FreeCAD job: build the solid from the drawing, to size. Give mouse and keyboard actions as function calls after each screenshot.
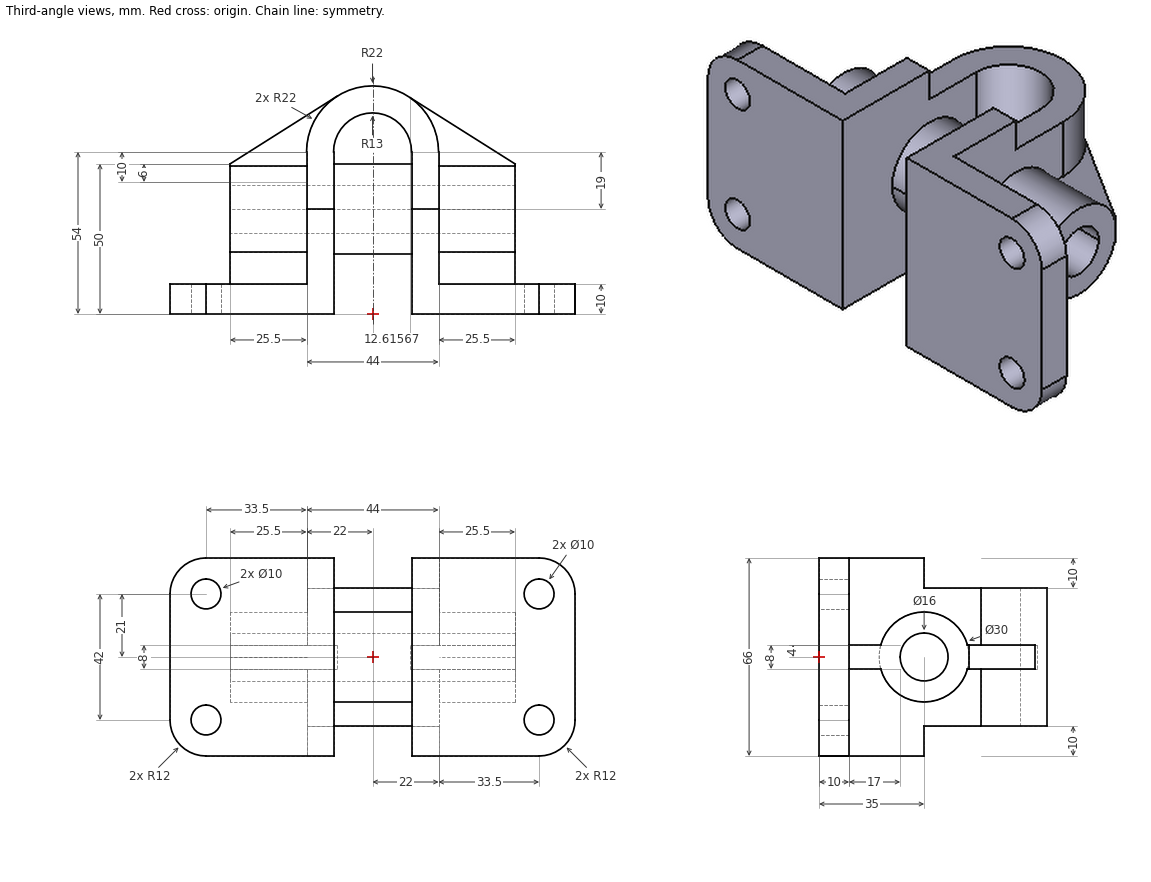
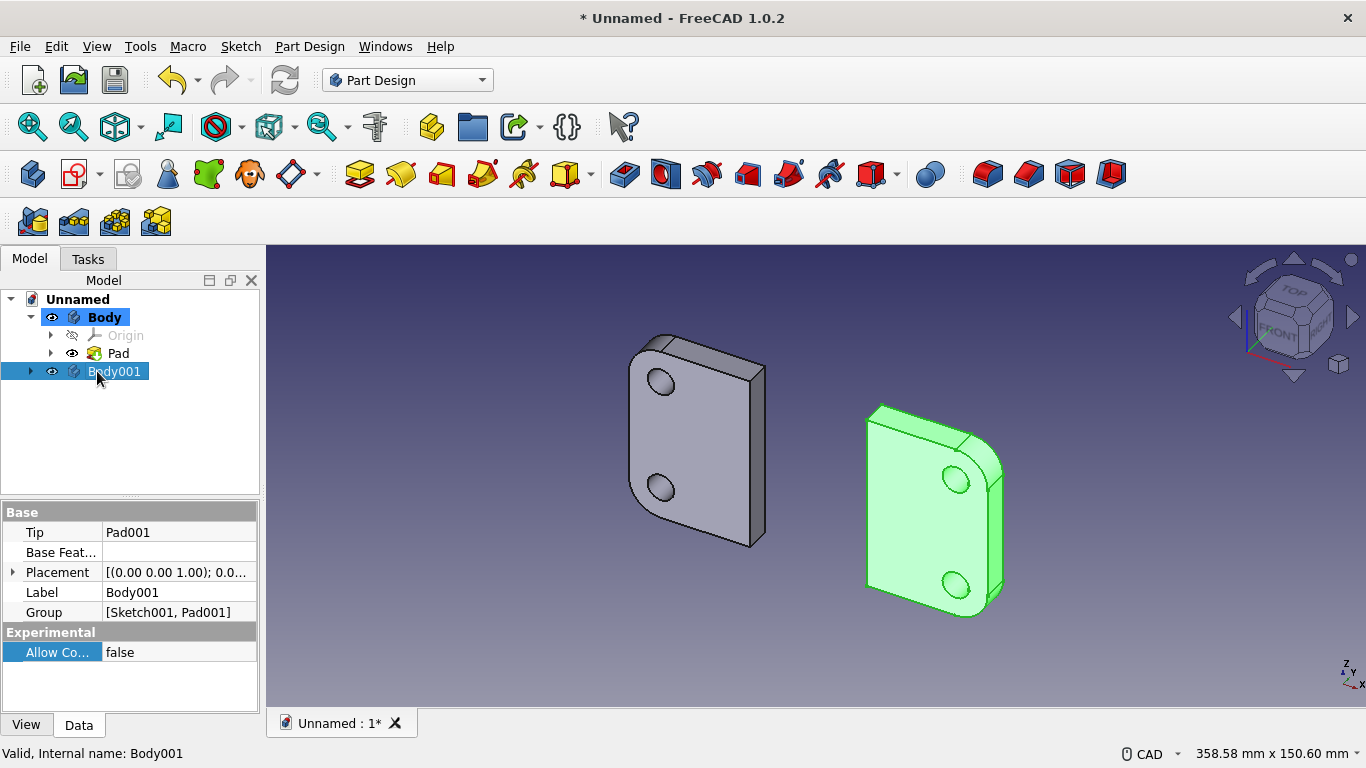
click(931, 174)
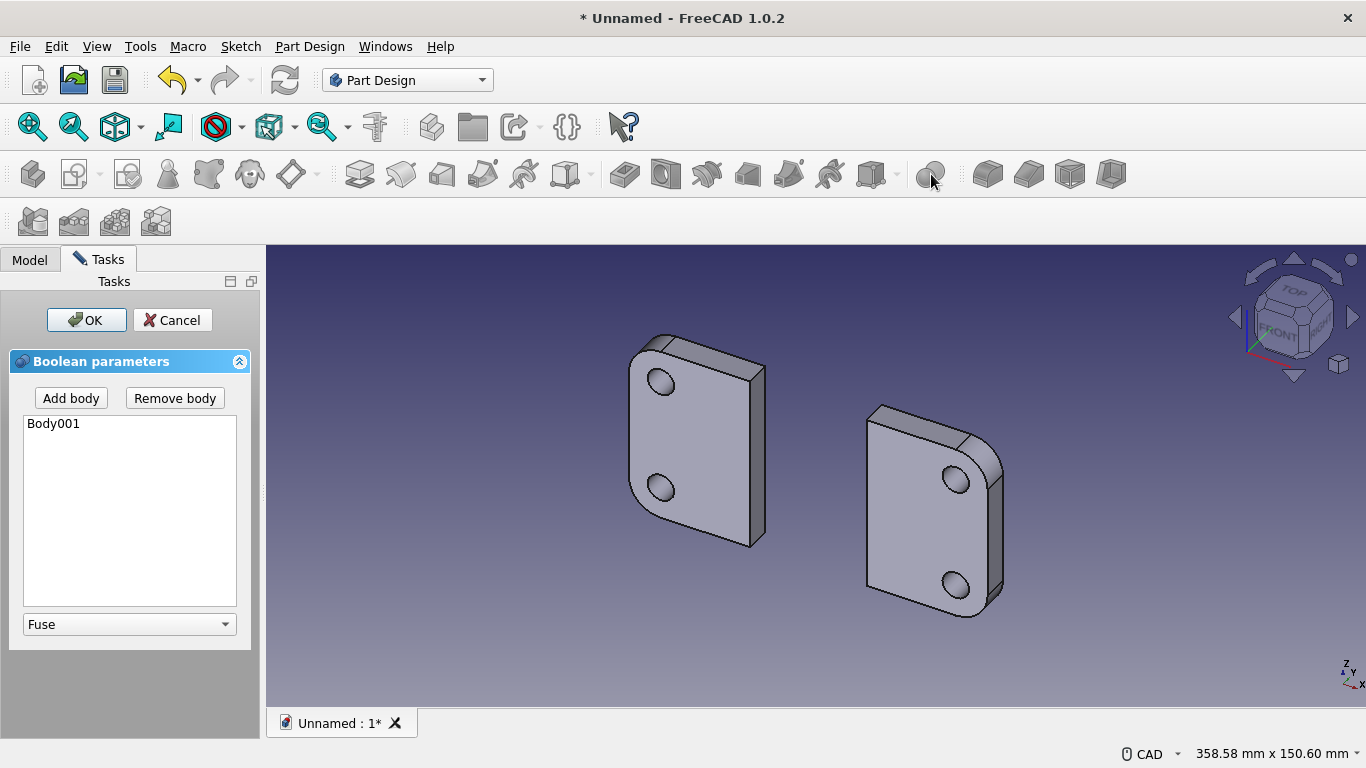
click(87, 320)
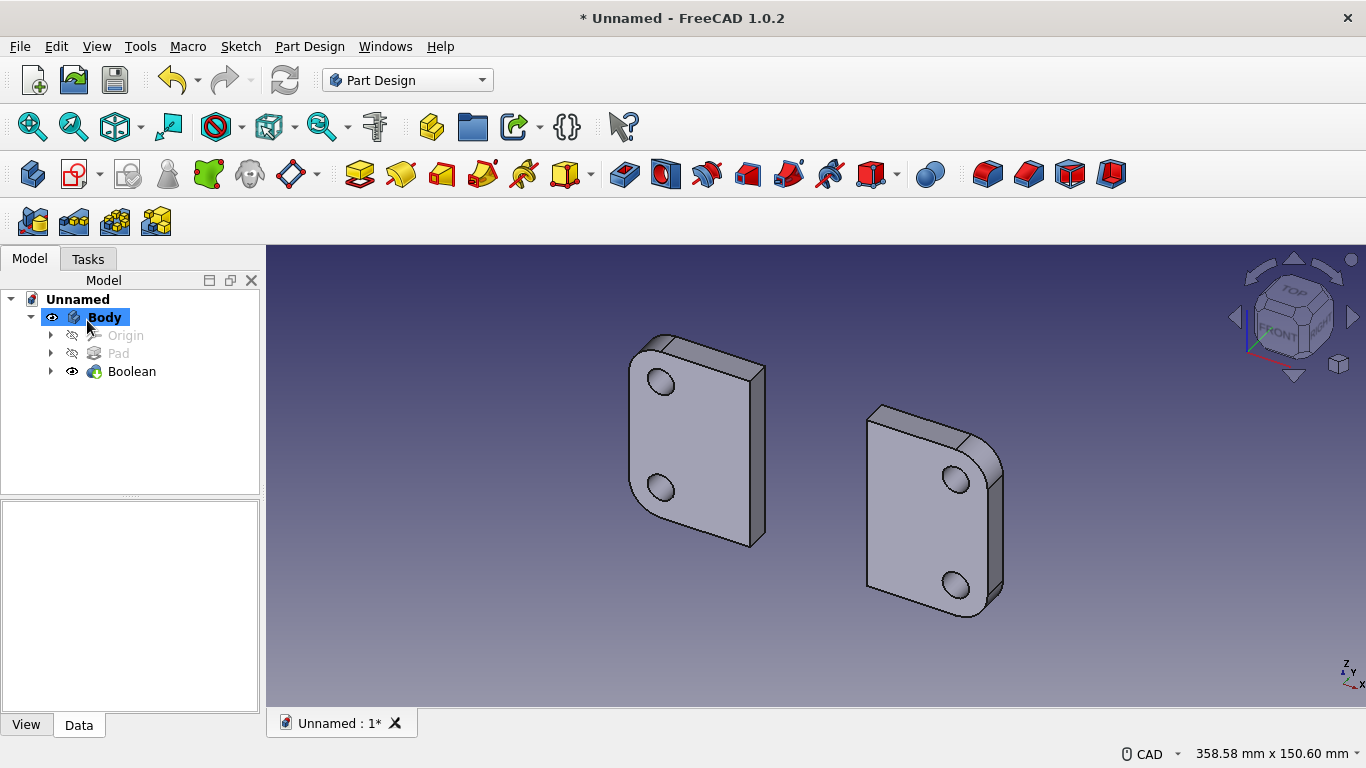
click(738, 366)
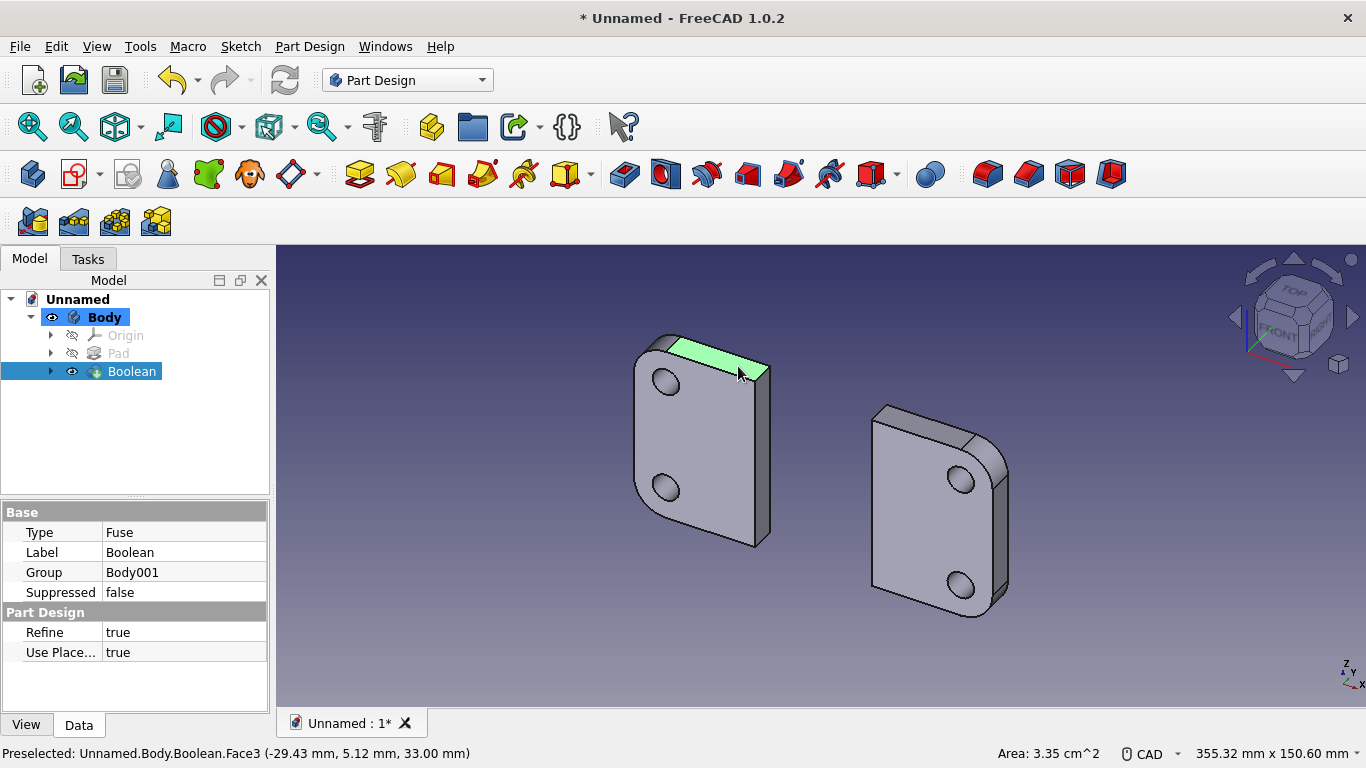
click(74, 174)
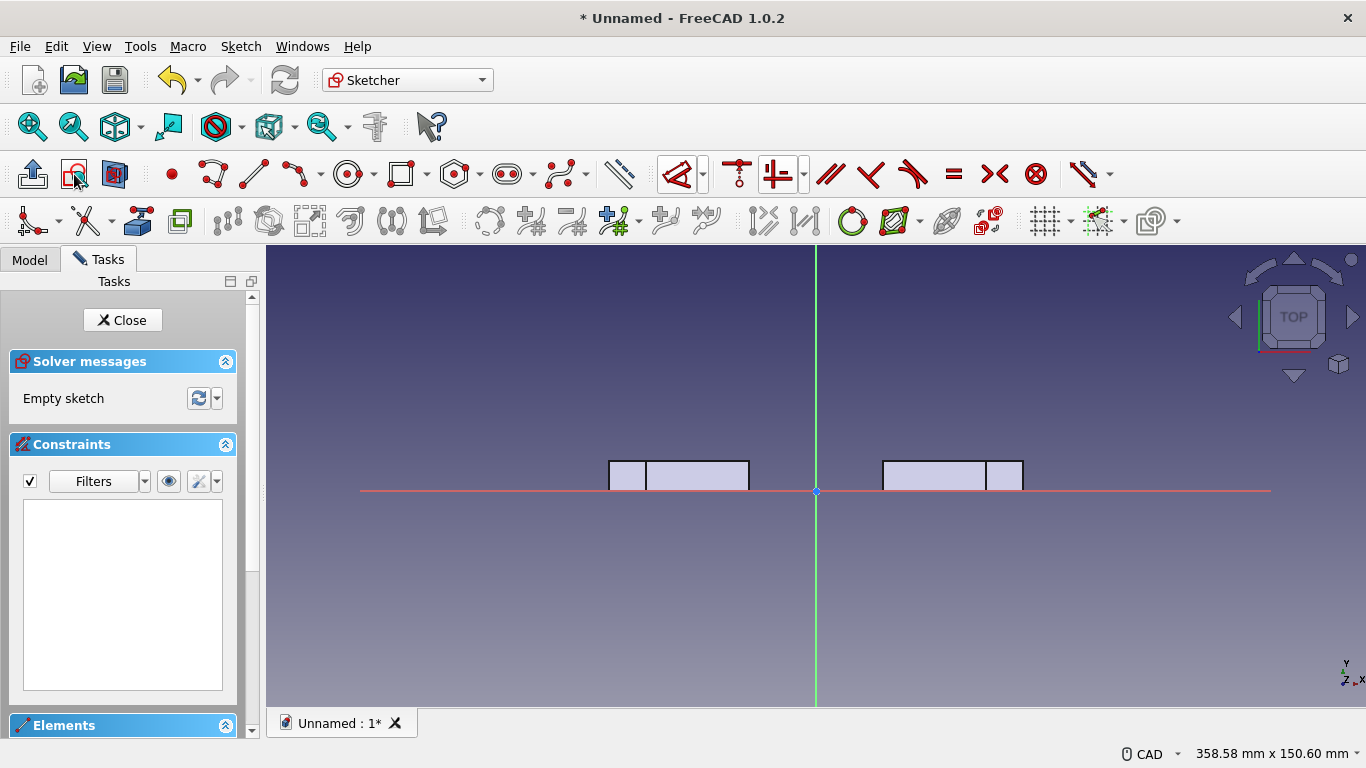
scroll(438, 679, down, 1)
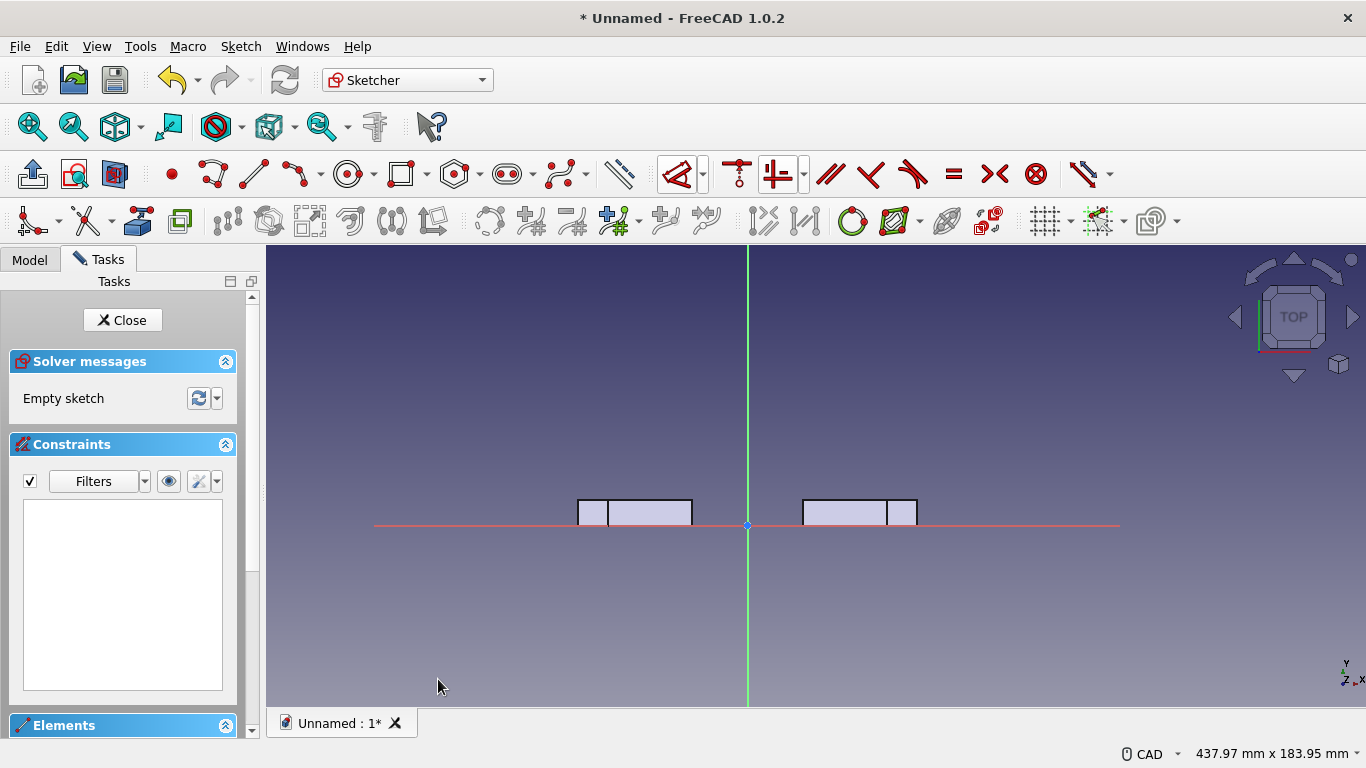
scroll(748, 337, up, 2)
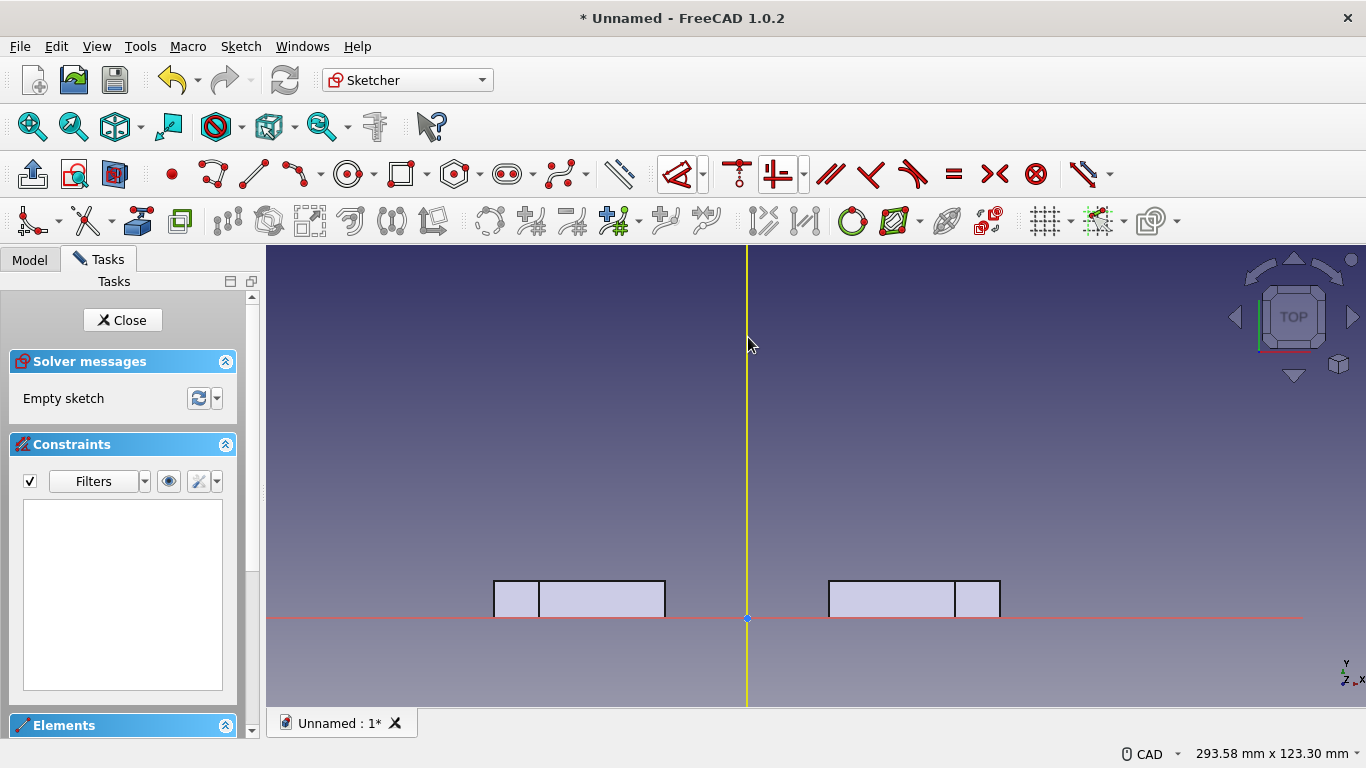
click(213, 174)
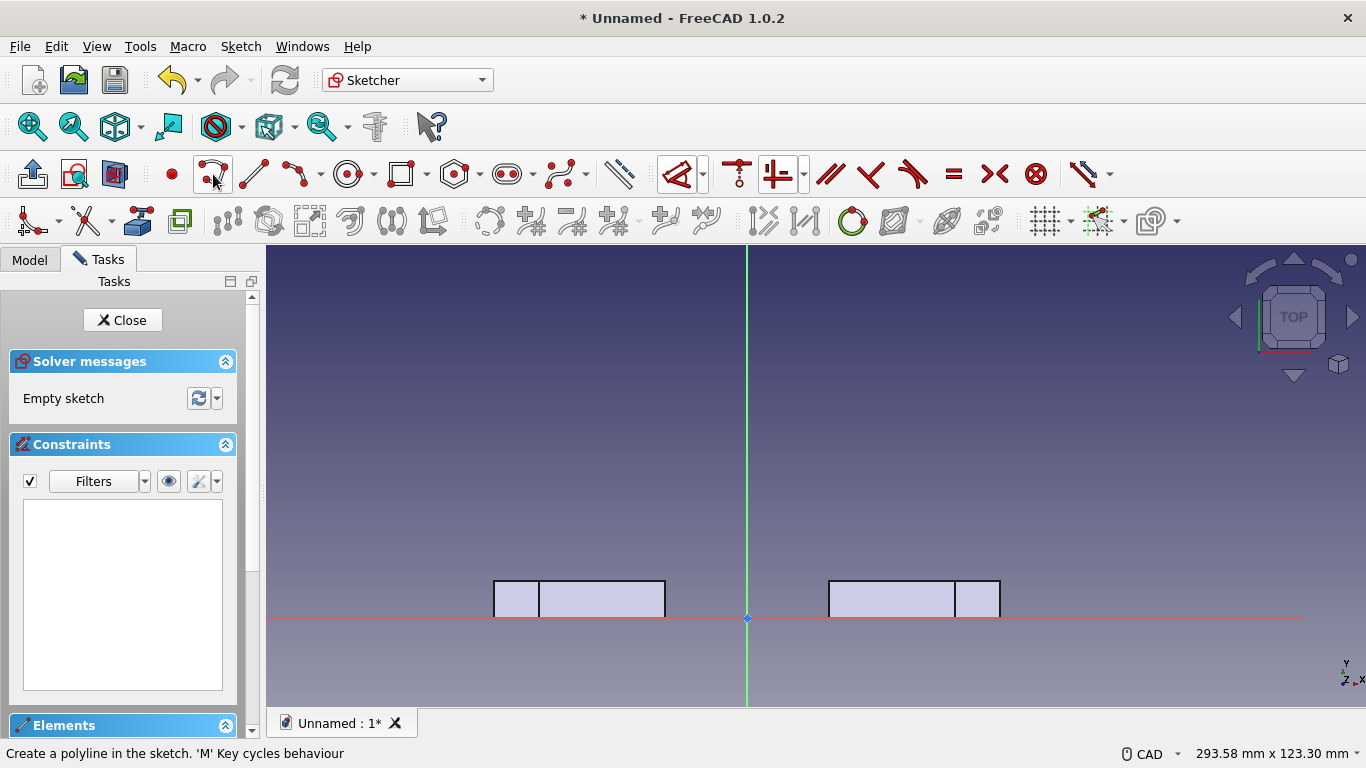
click(665, 416)
click(665, 618)
click(698, 609)
click(698, 416)
right_click(698, 416)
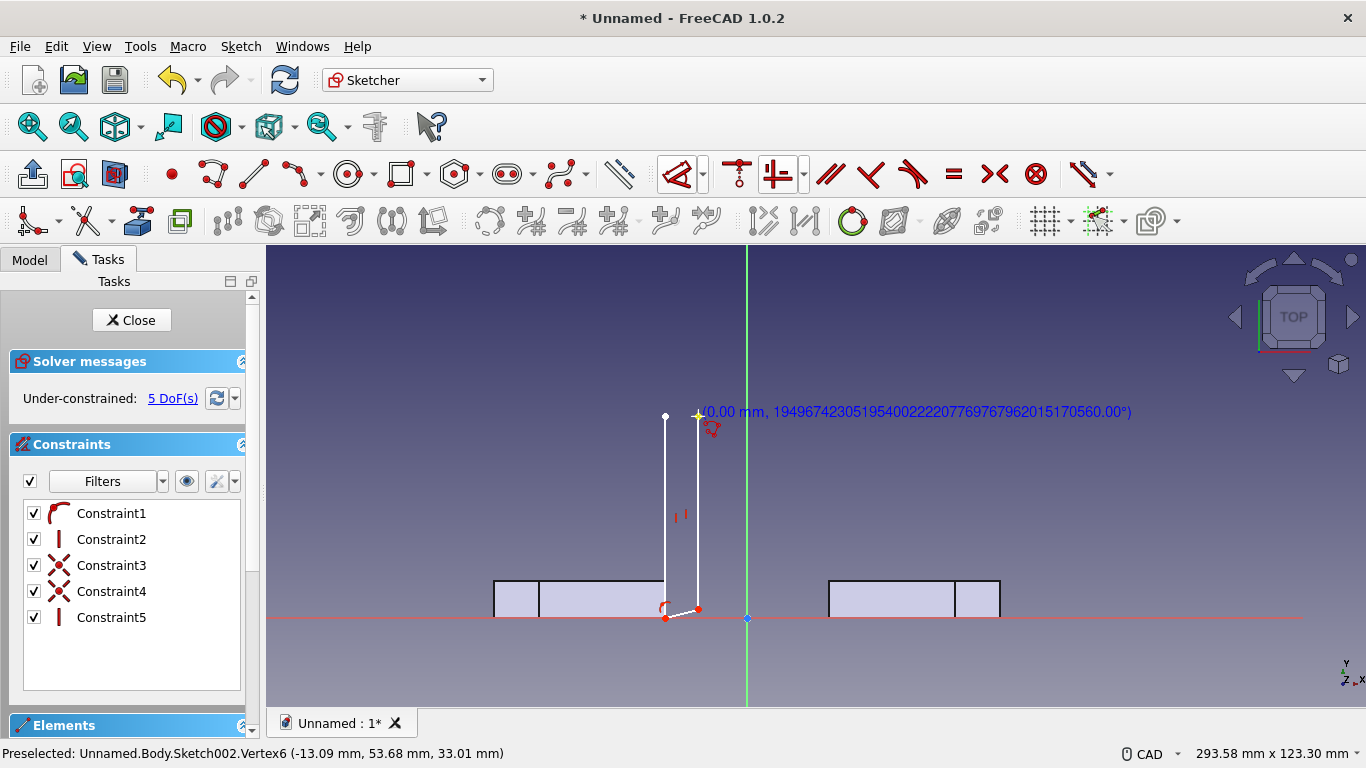
click(796, 416)
click(796, 618)
click(829, 609)
click(829, 416)
right_click(829, 416)